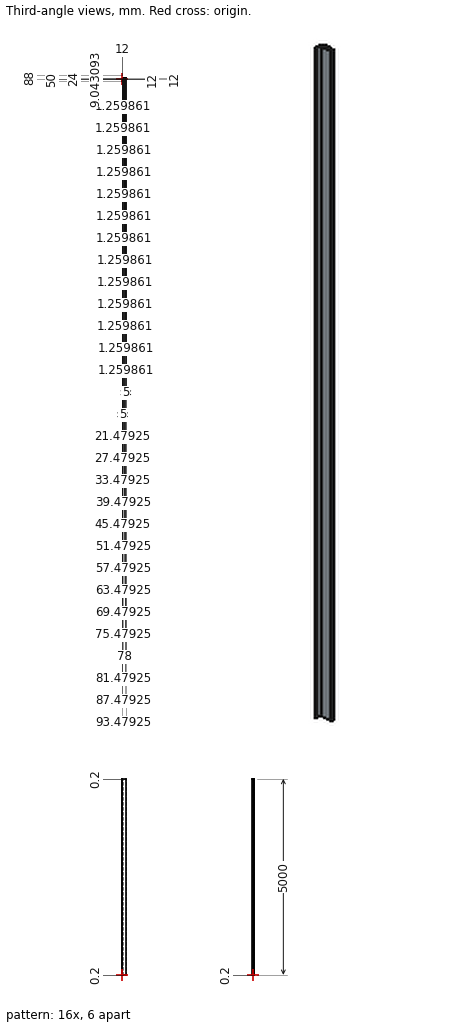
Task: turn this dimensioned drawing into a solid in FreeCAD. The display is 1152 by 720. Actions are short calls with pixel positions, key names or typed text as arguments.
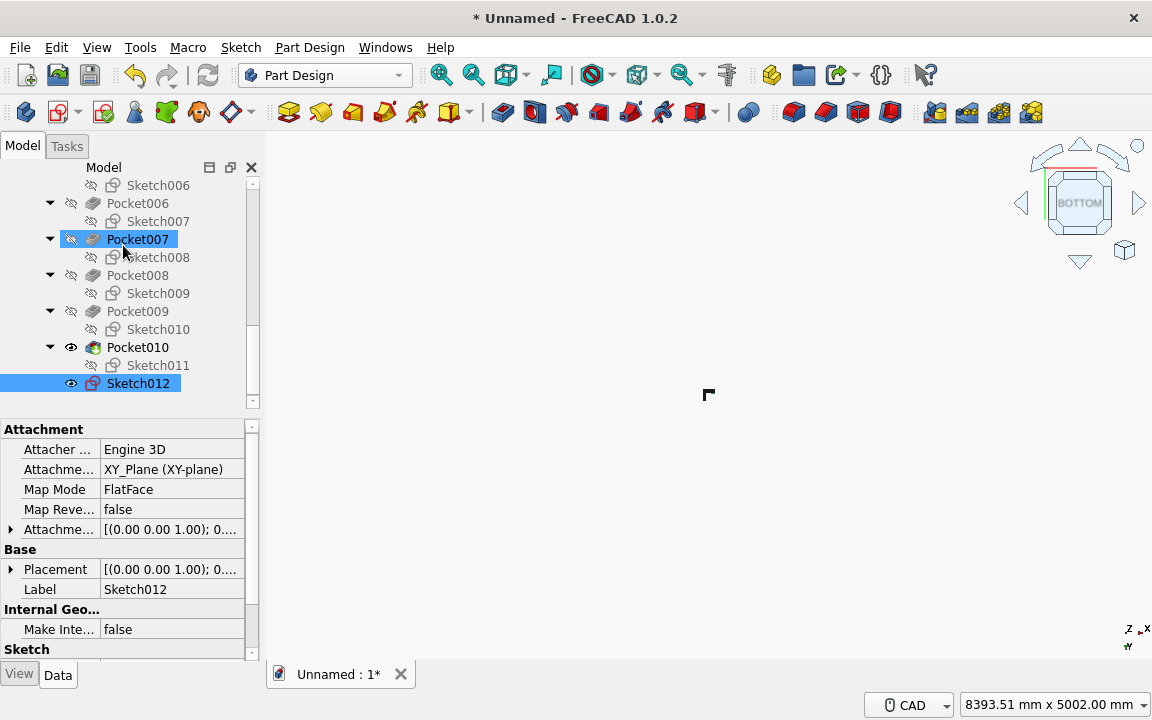
click(504, 112)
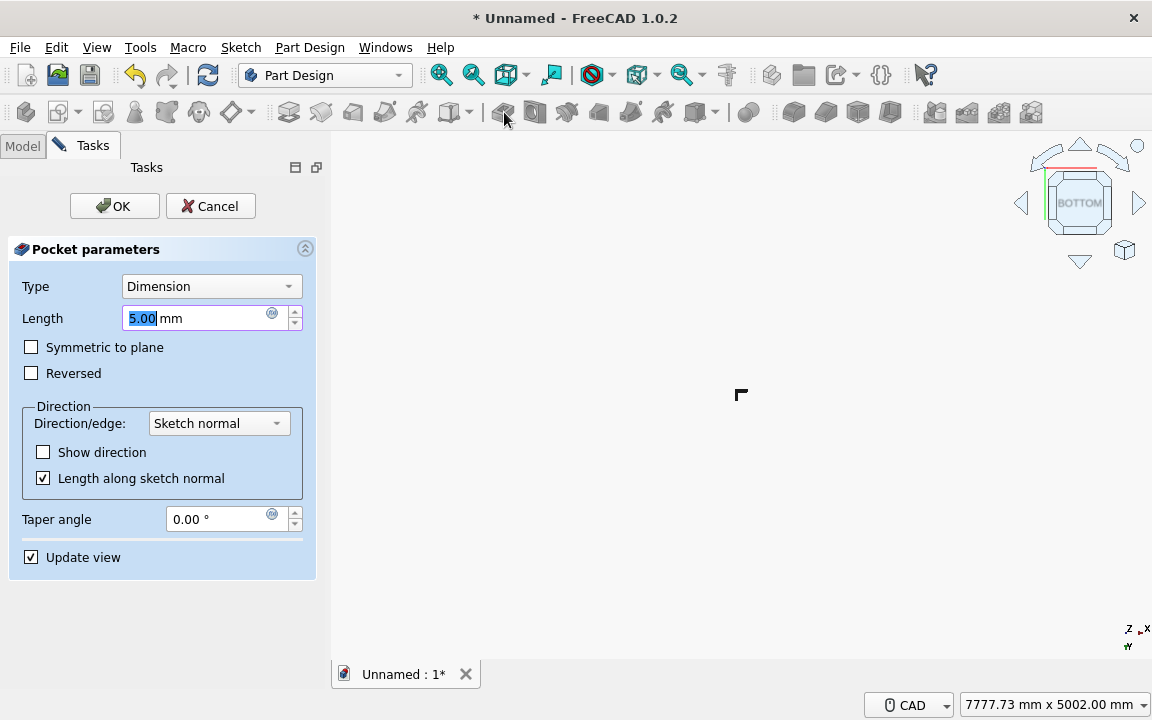
text(0.2)
key(Tab)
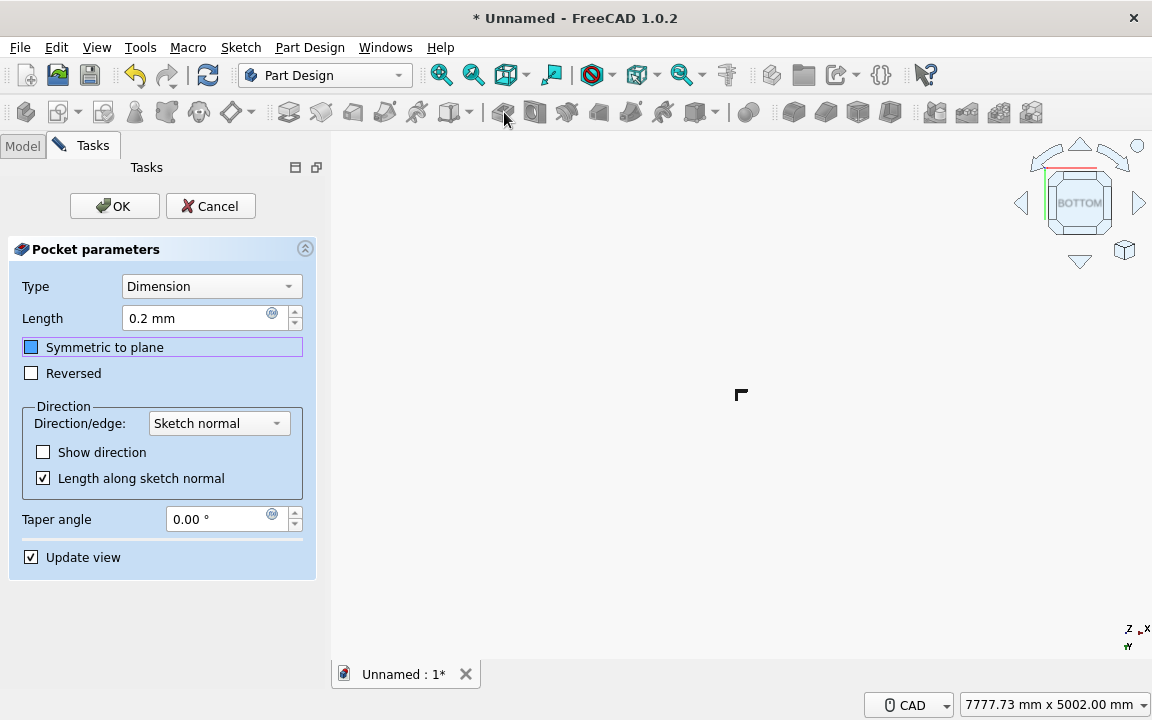
click(30, 373)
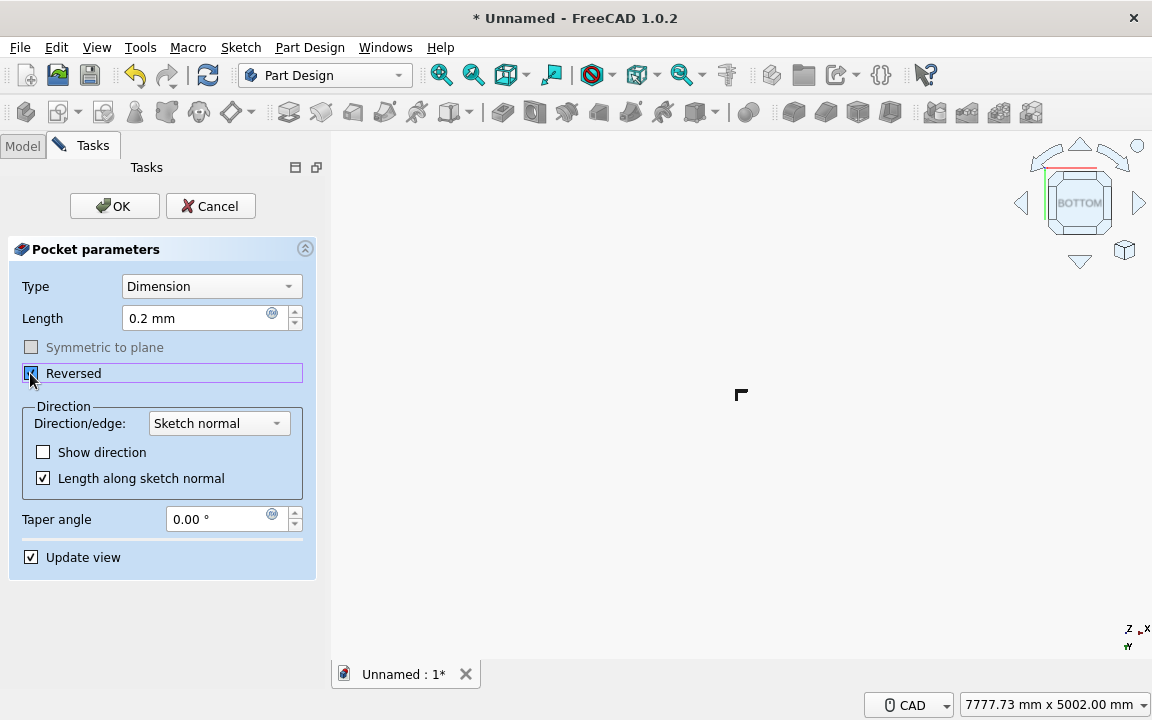
click(115, 206)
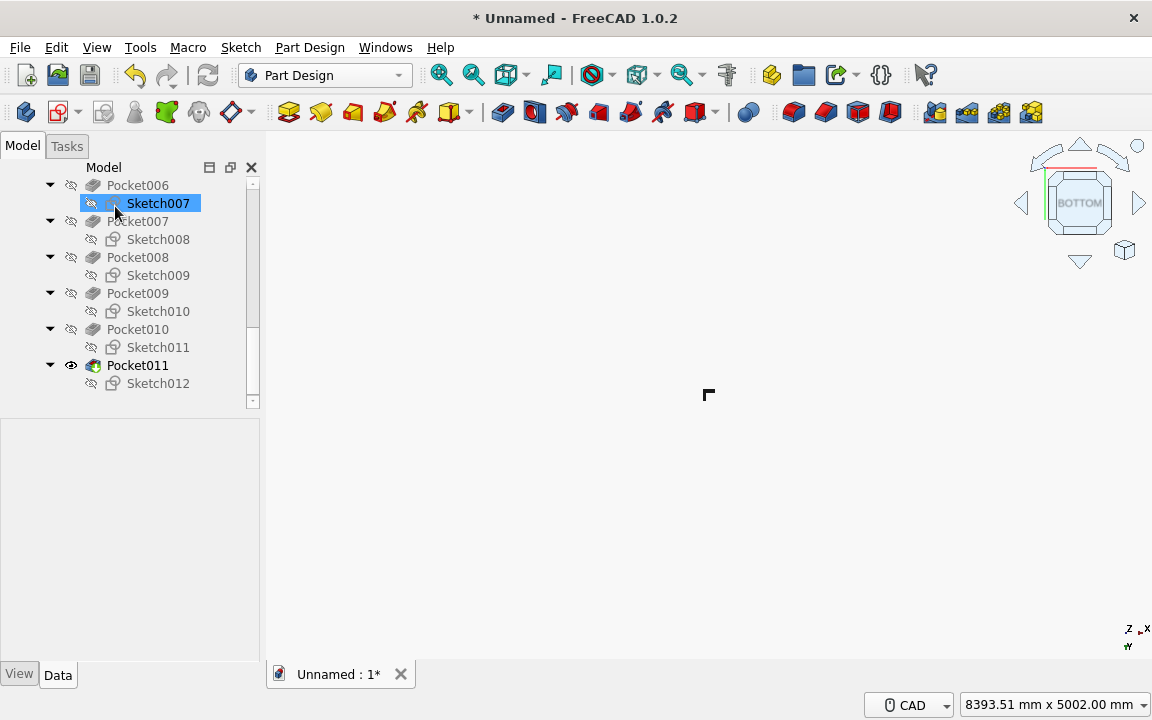
click(442, 76)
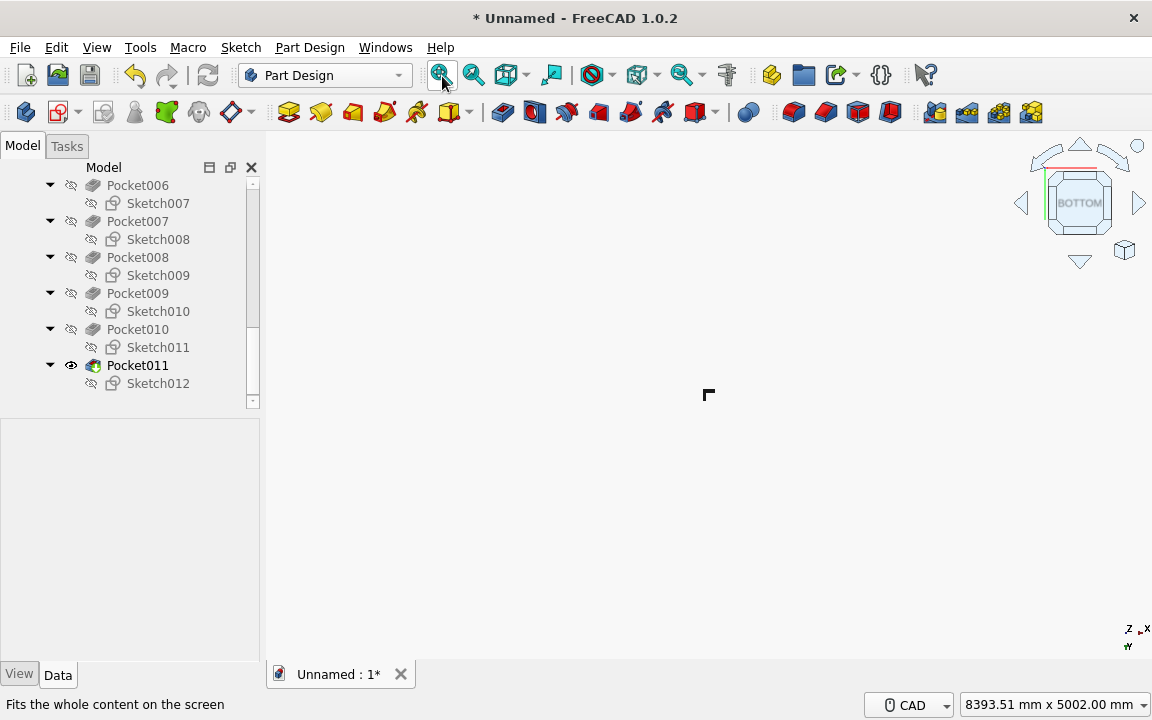
scroll(712, 389, up, 14)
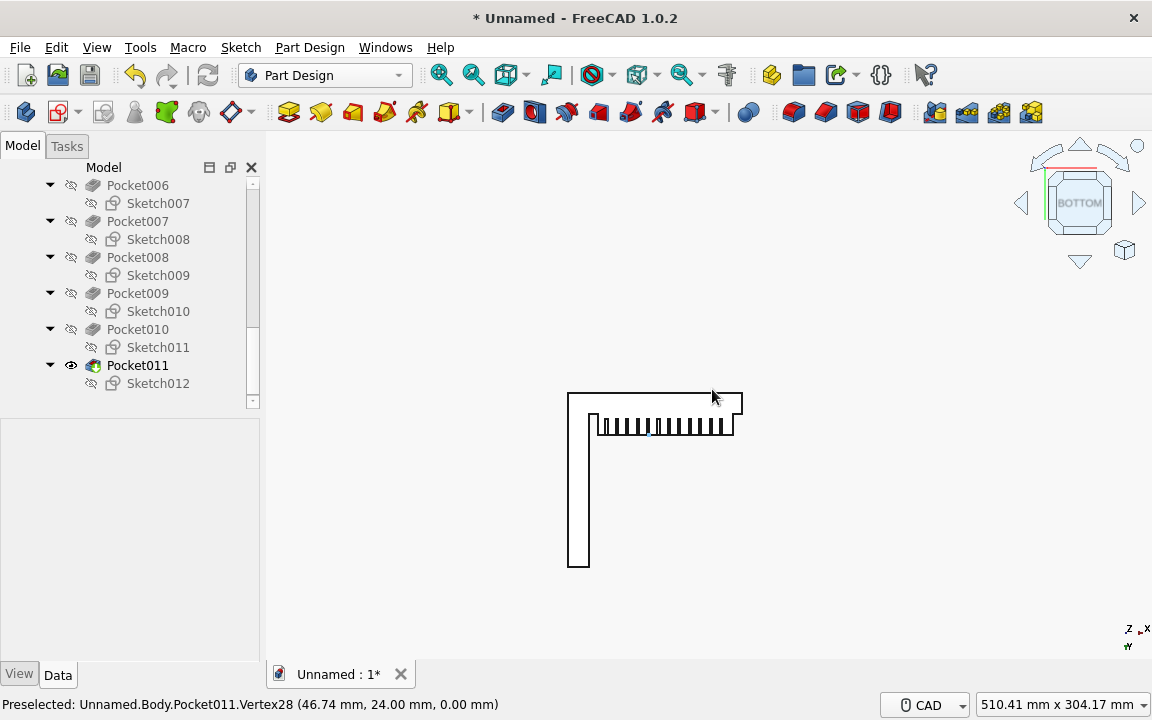
click(704, 405)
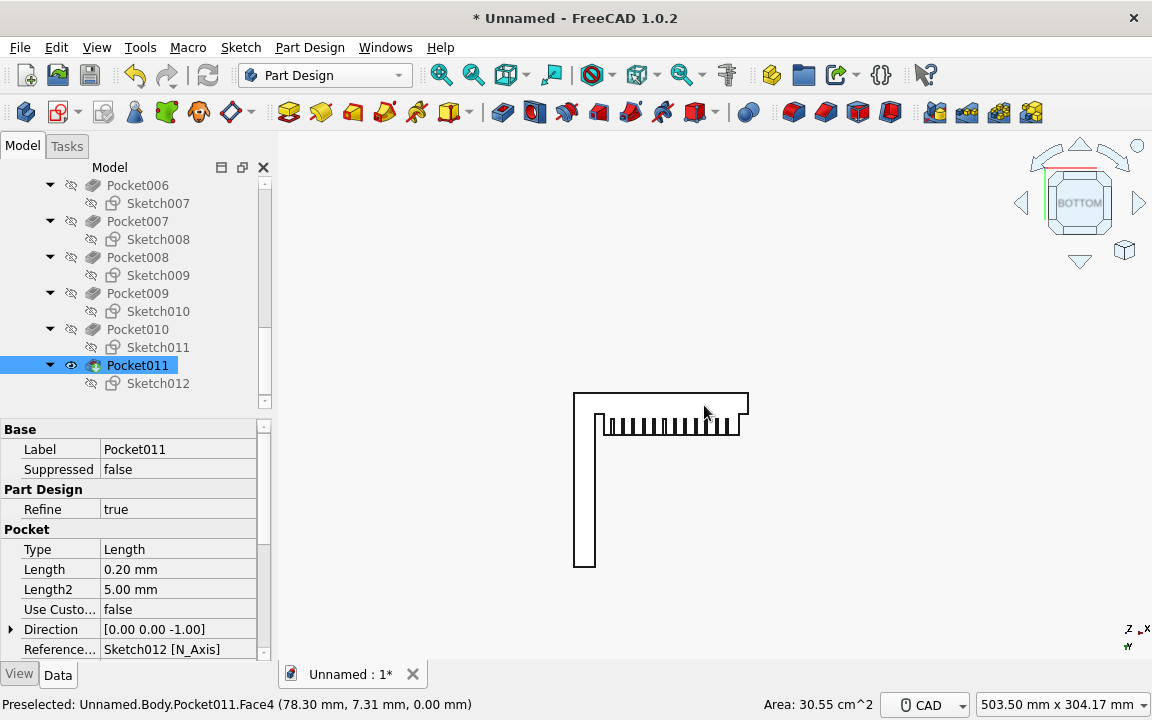
click(58, 112)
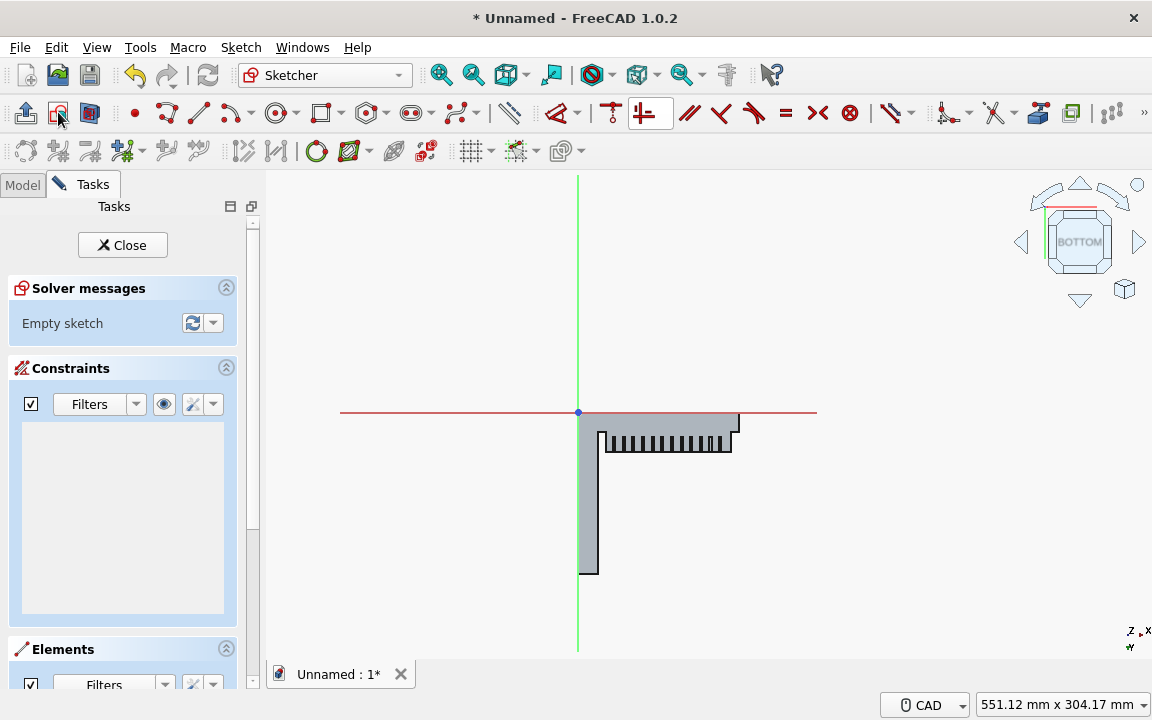
scroll(734, 446, up, 15)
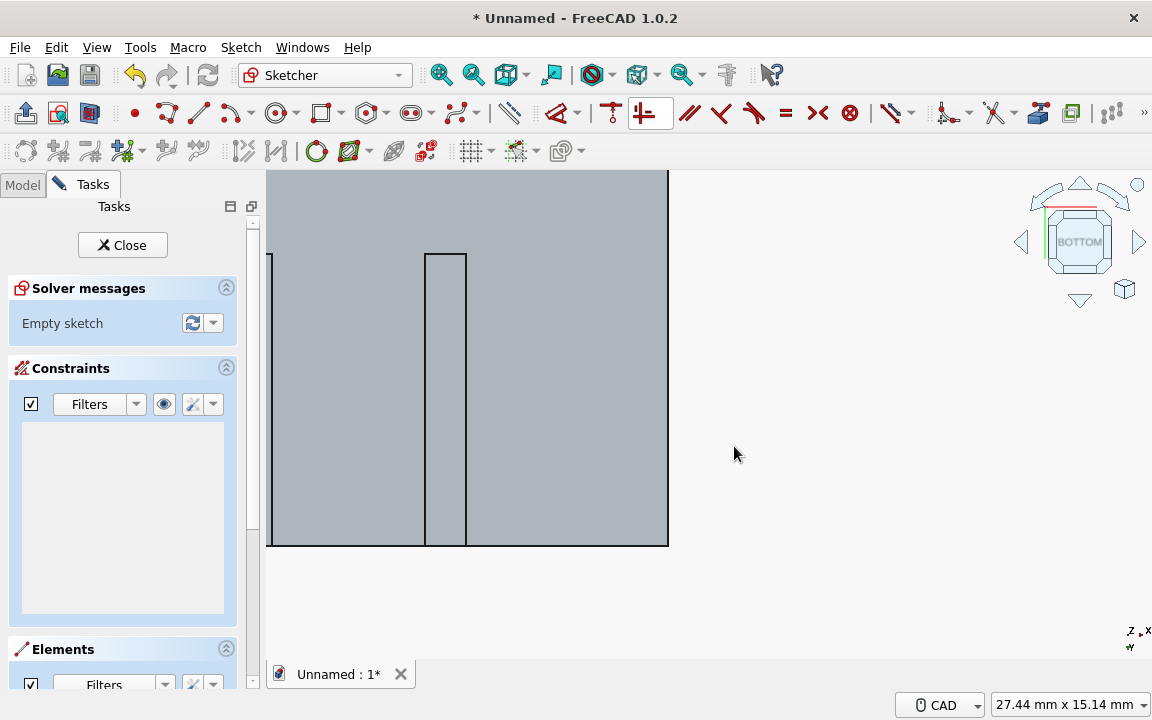
click(322, 114)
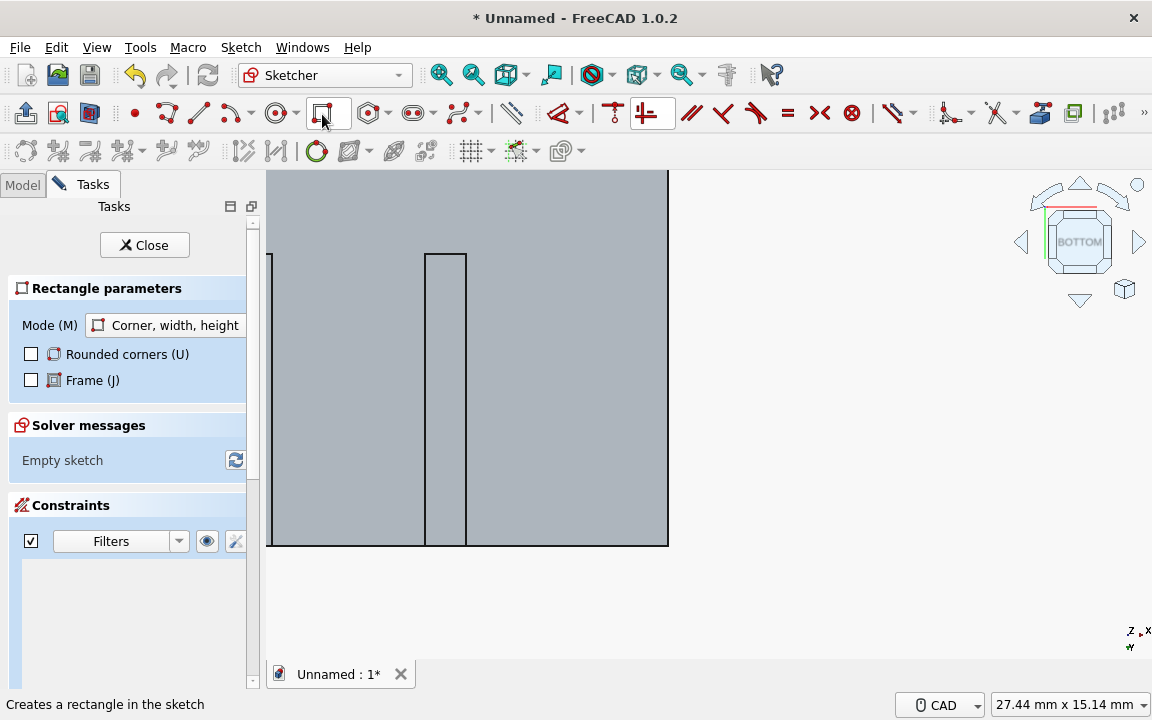
click(619, 254)
click(660, 546)
key(Escape)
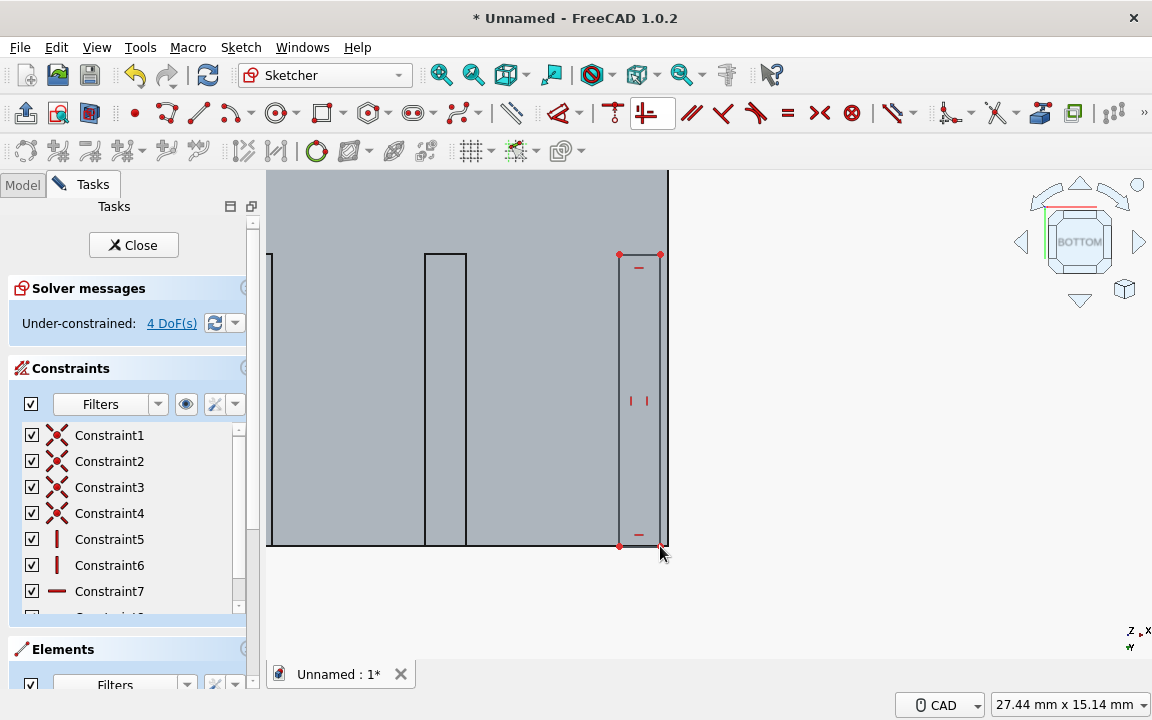
click(558, 114)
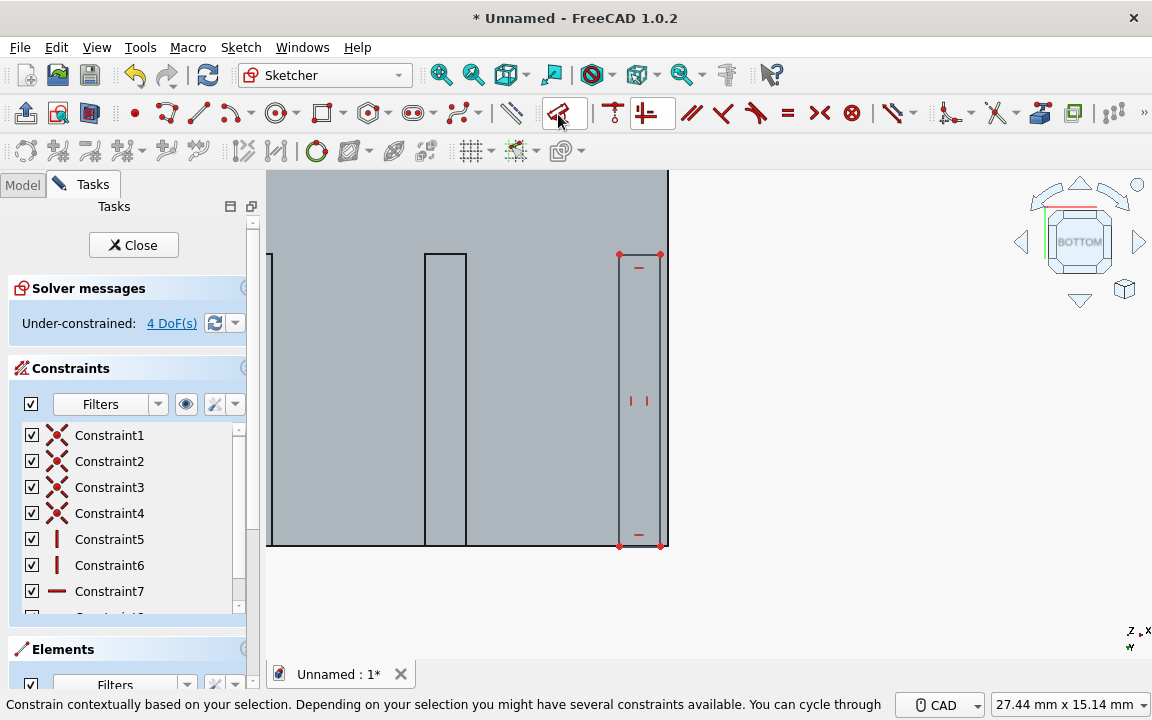
click(619, 547)
click(677, 373)